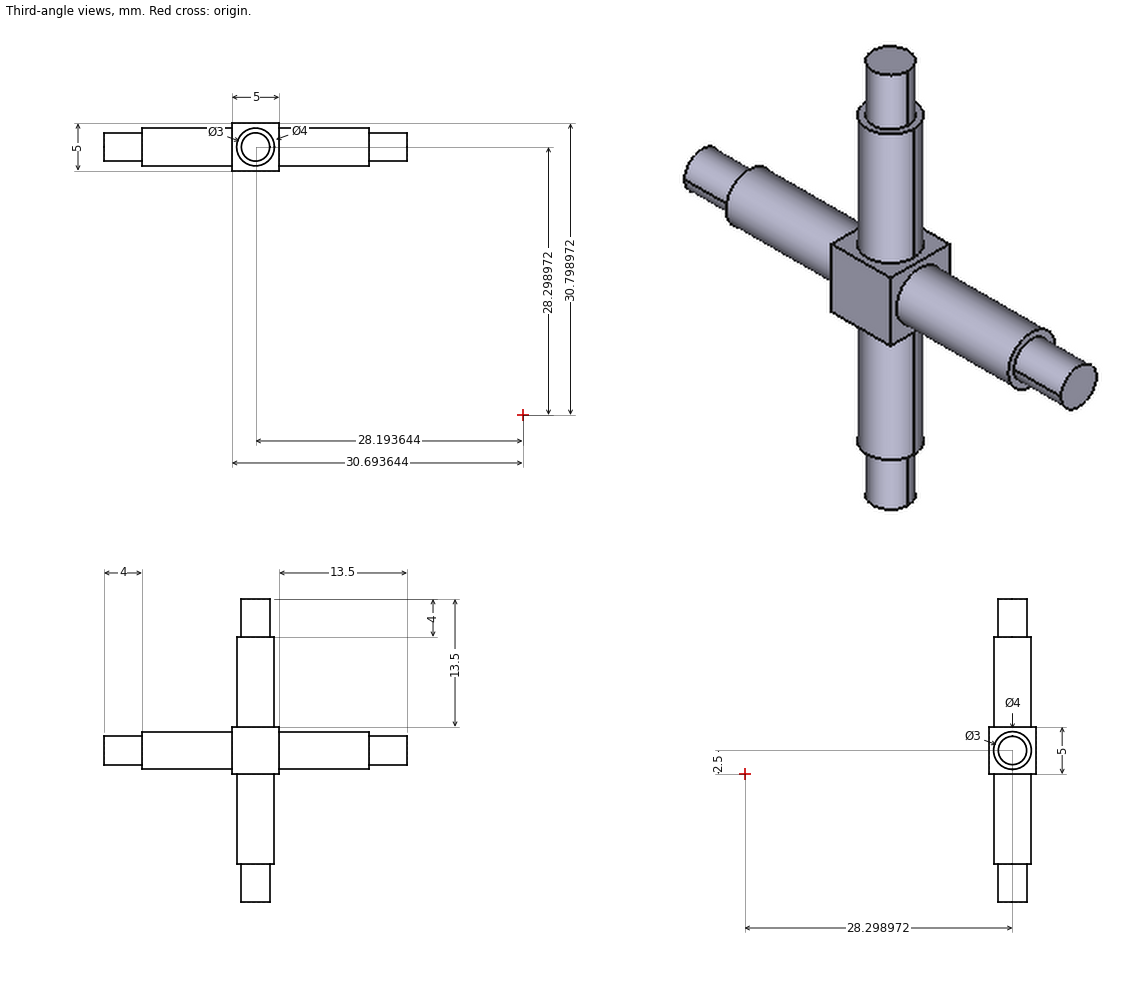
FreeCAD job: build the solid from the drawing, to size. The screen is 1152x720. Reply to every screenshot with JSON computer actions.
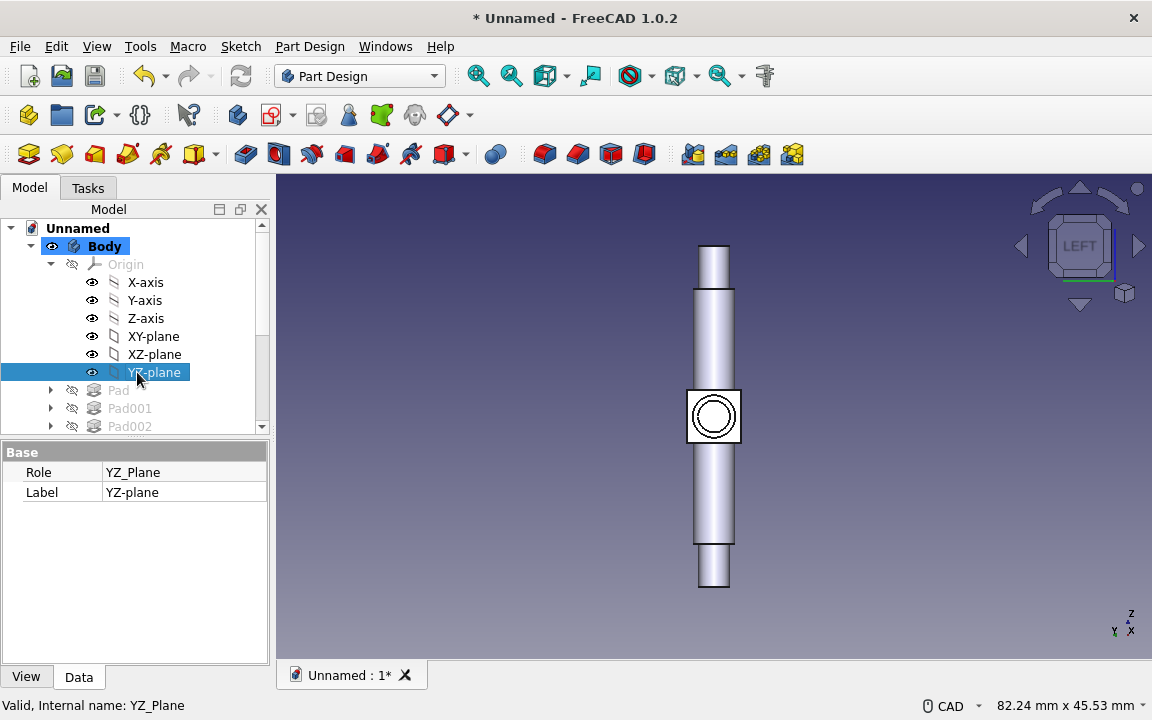
{"action": "left_click", "coordinate": [448, 116]}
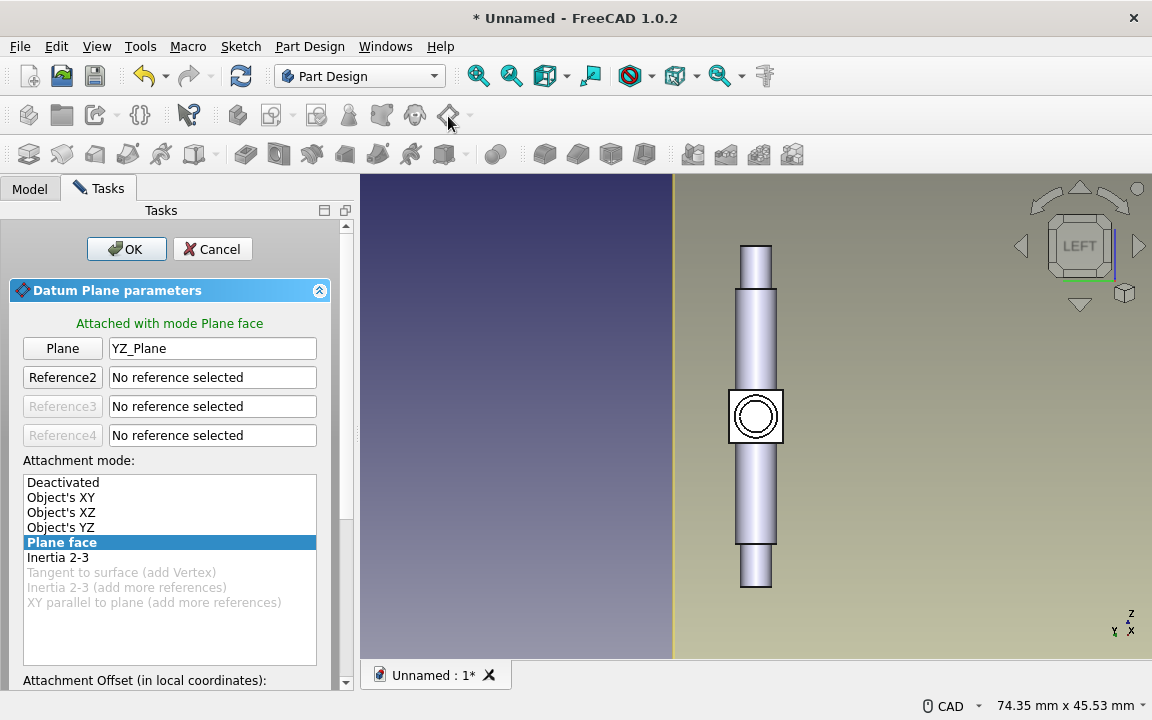
{"action": "scroll", "coordinate": [346, 455], "scroll_direction": "down", "scroll_amount": 3}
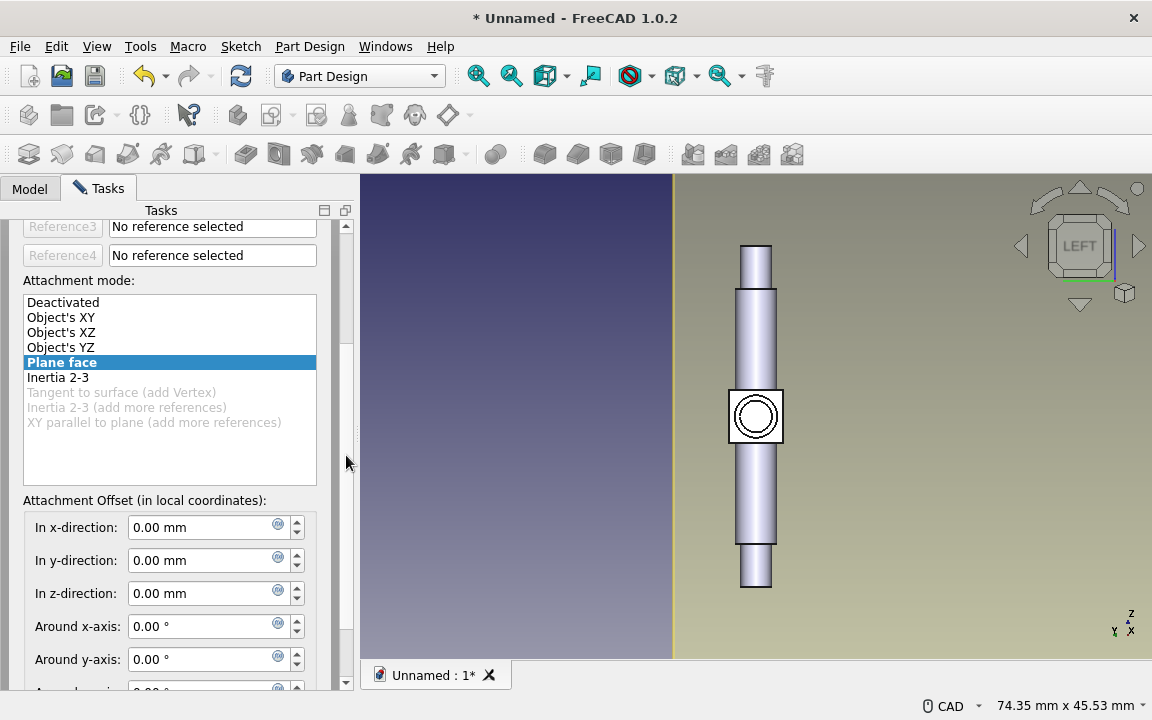
{"action": "triple_click", "coordinate": [210, 594]}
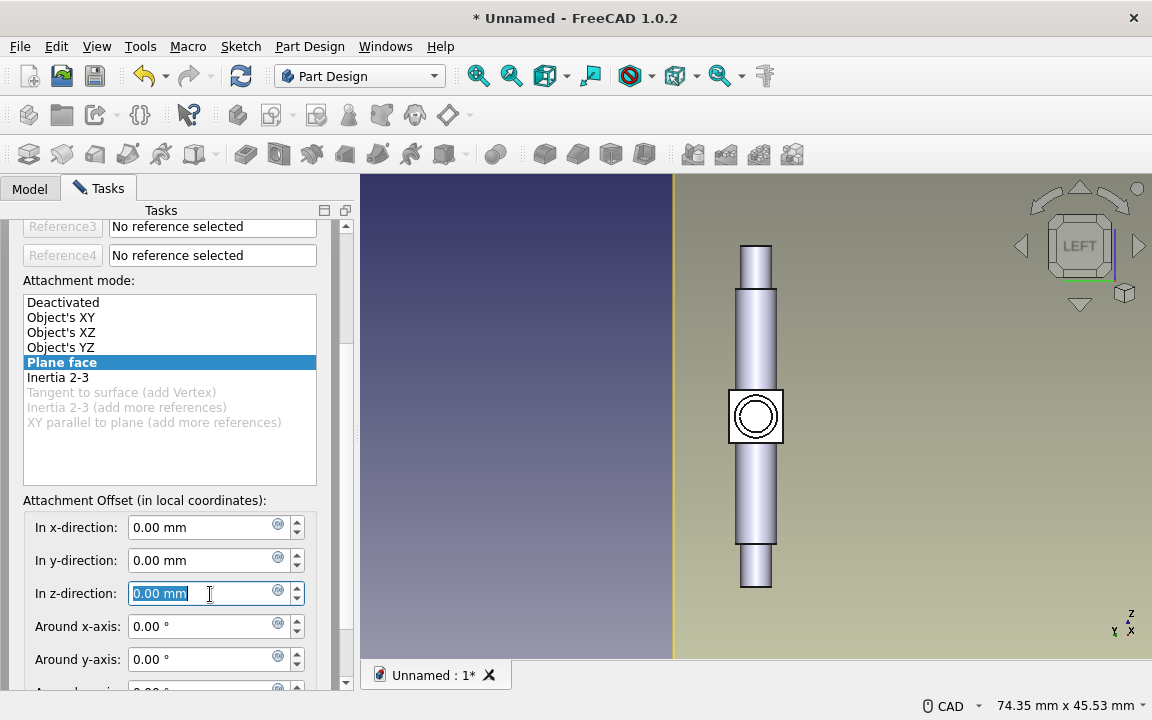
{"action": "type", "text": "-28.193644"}
{"action": "key", "text": "Tab"}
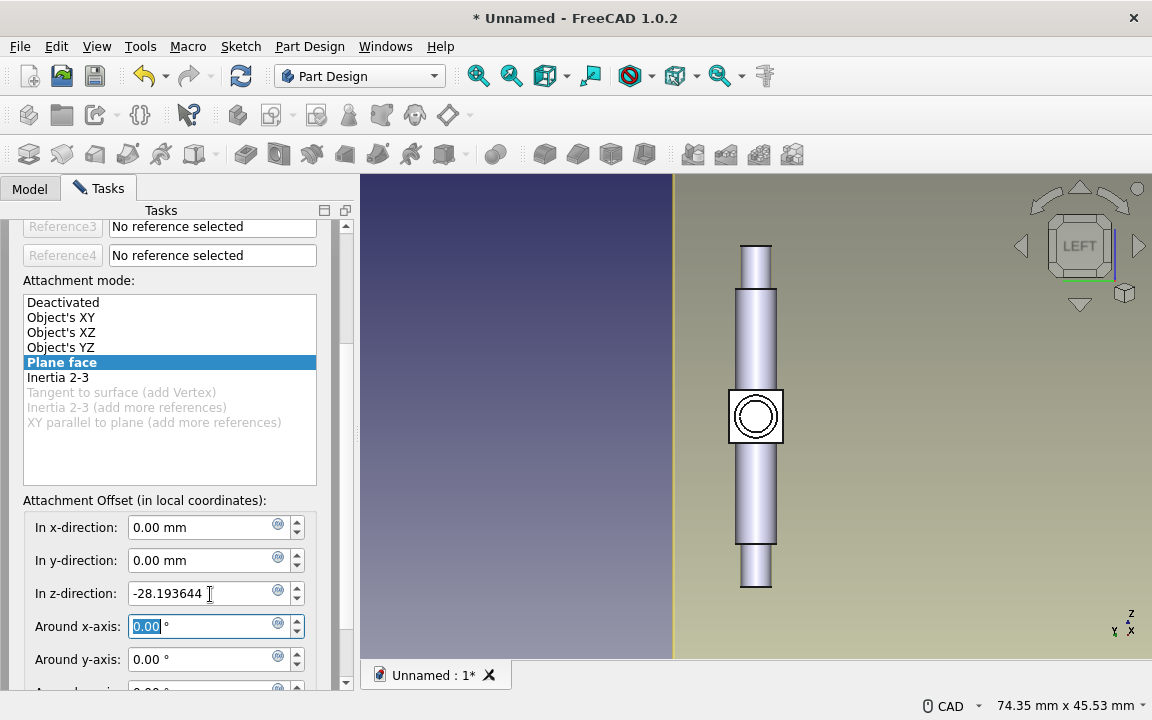
{"action": "scroll", "coordinate": [346, 455], "scroll_direction": "up", "scroll_amount": 4}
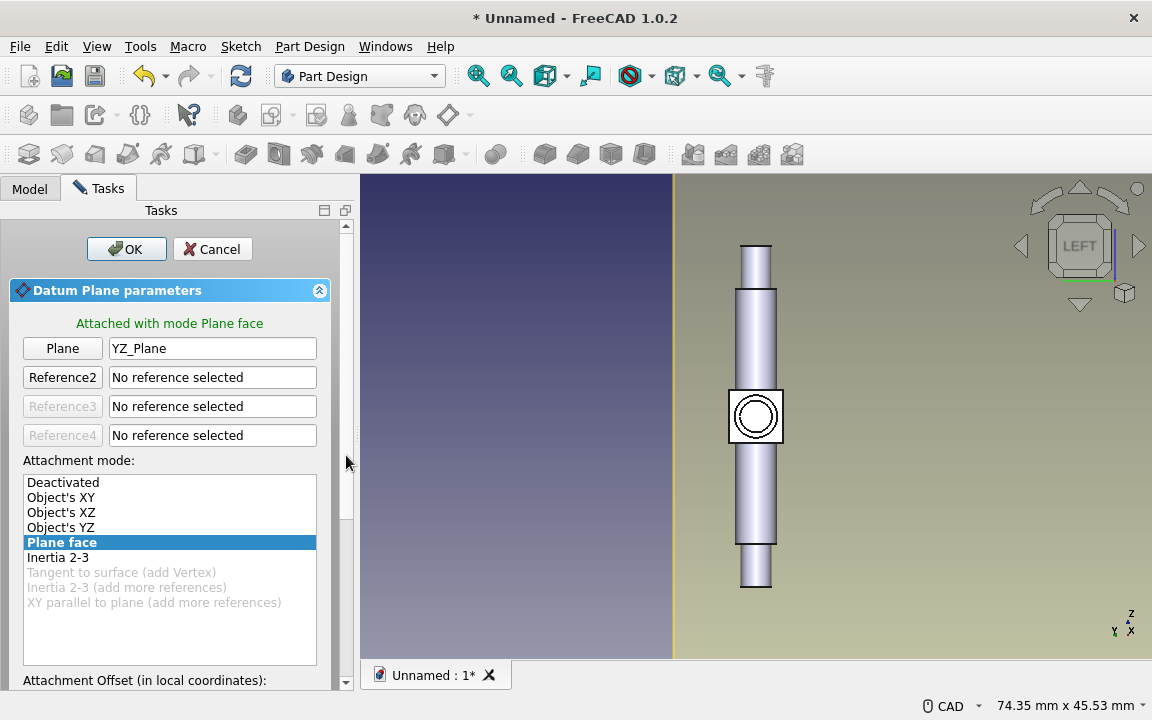
{"action": "left_click", "coordinate": [127, 249]}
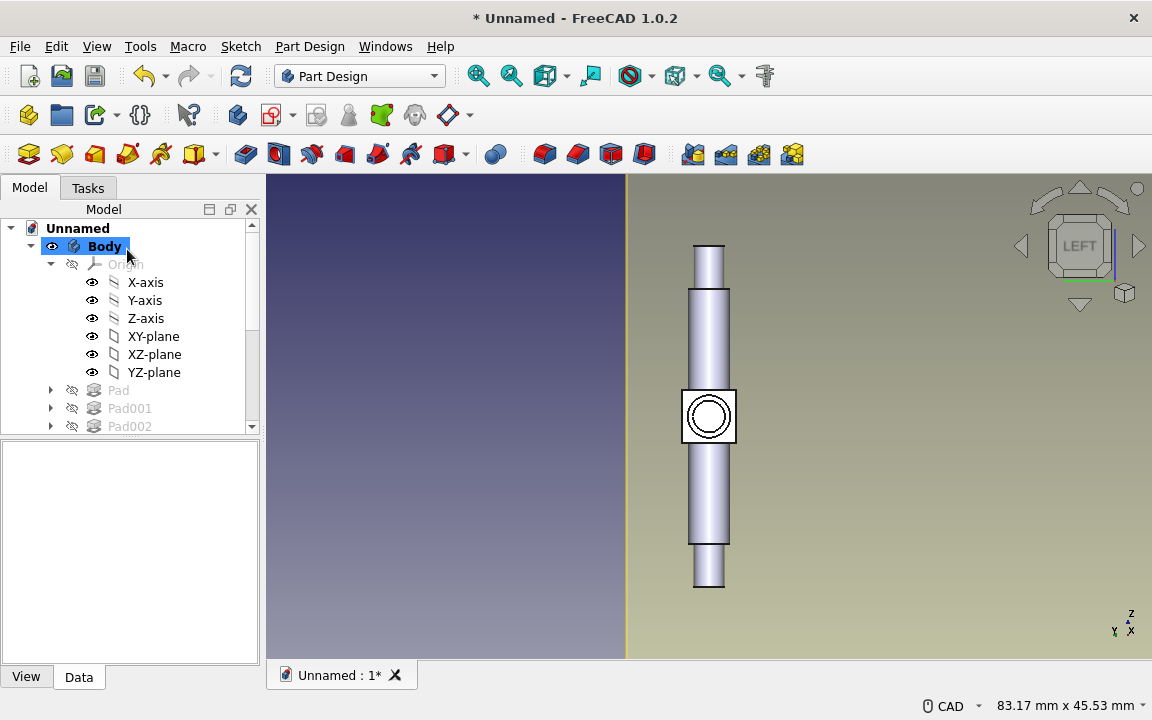
{"action": "scroll", "coordinate": [101, 332], "scroll_direction": "down", "scroll_amount": 3}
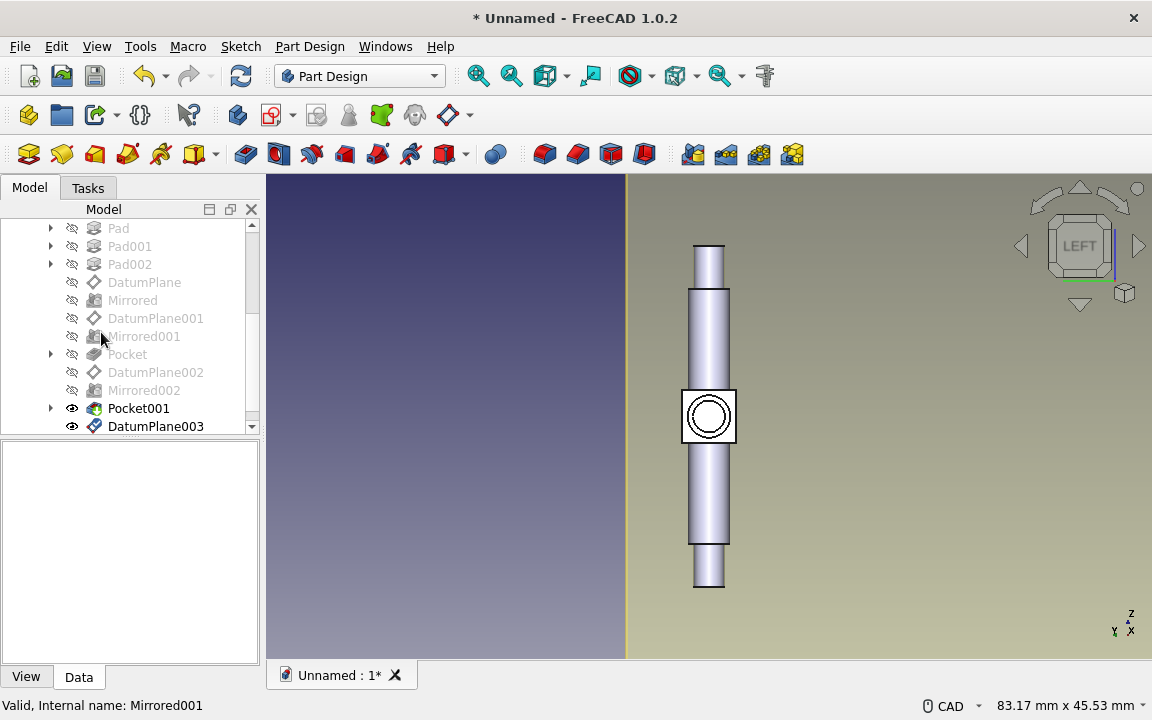
{"action": "left_click", "coordinate": [117, 408]}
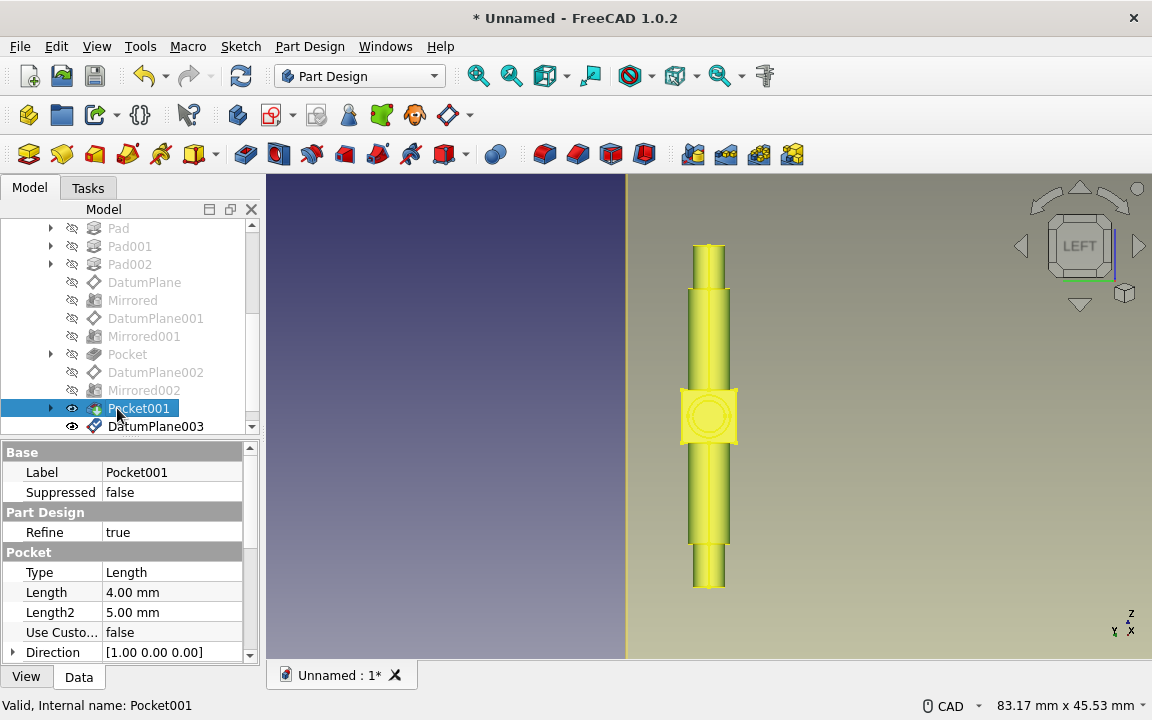
{"action": "left_click", "coordinate": [693, 154]}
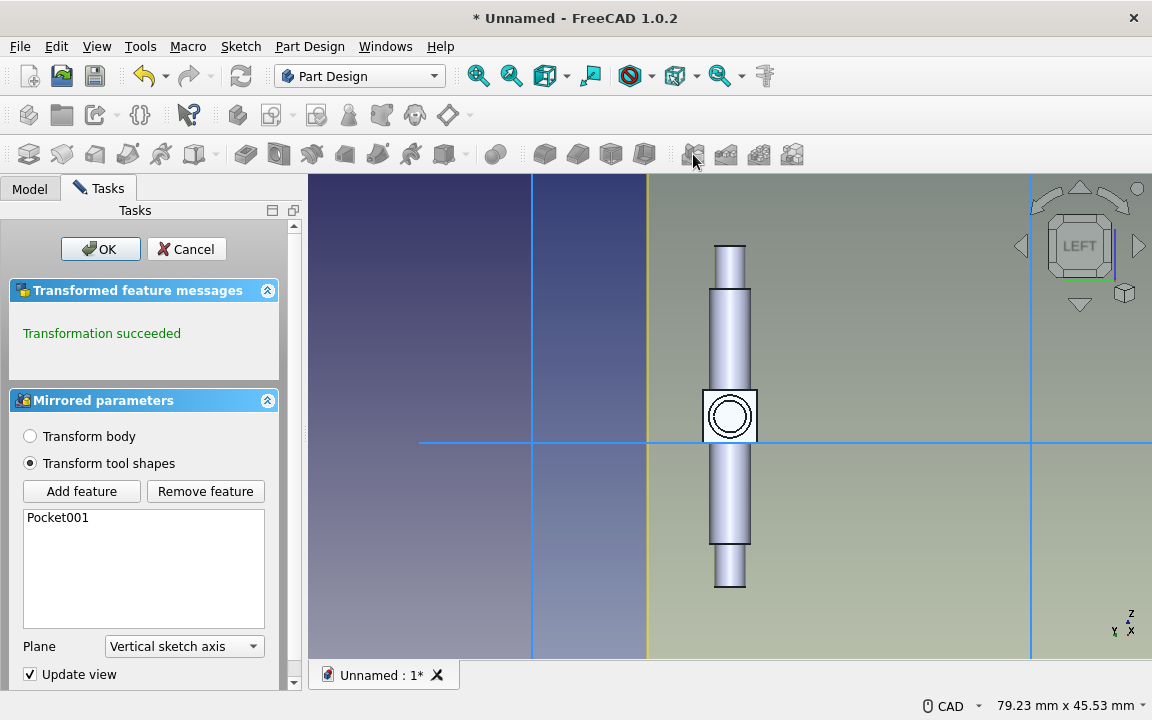
{"action": "left_click", "coordinate": [185, 646]}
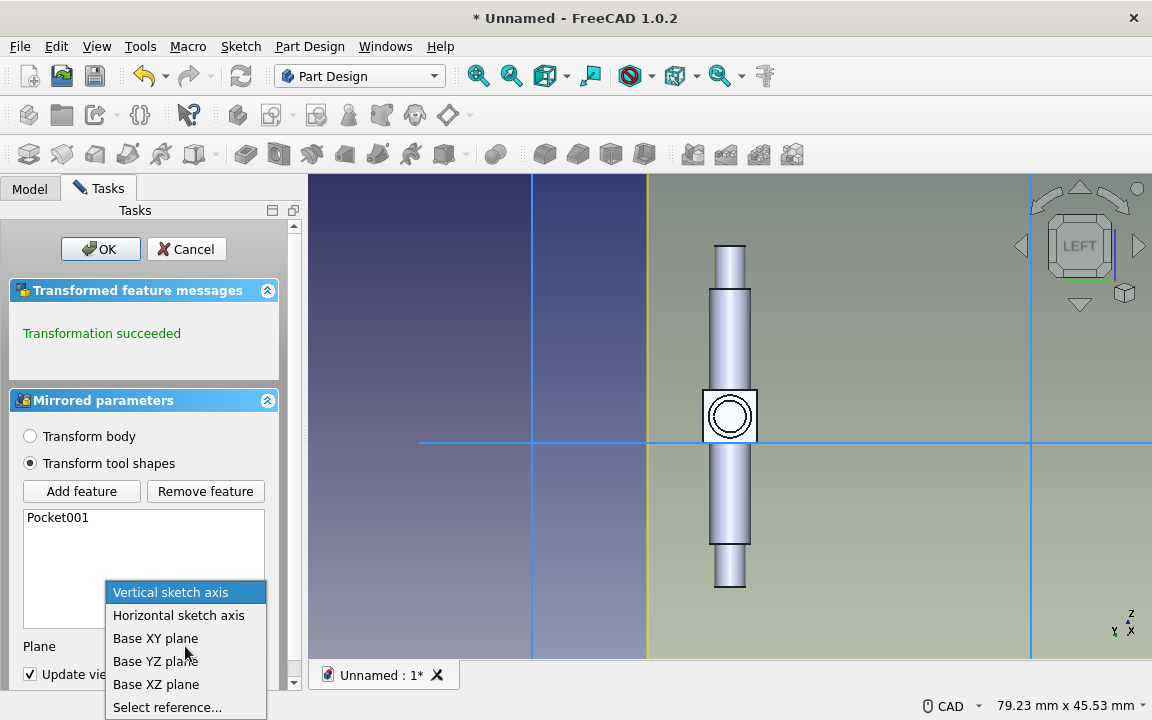
{"action": "left_click", "coordinate": [184, 708]}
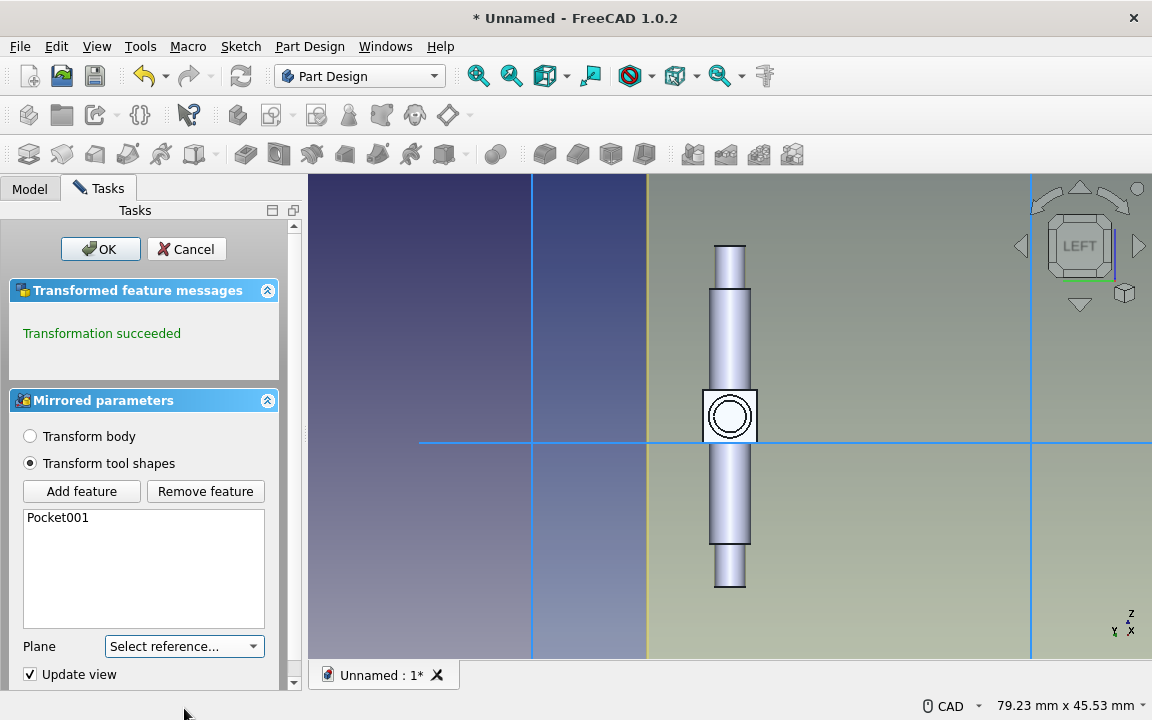
{"action": "left_click", "coordinate": [30, 188]}